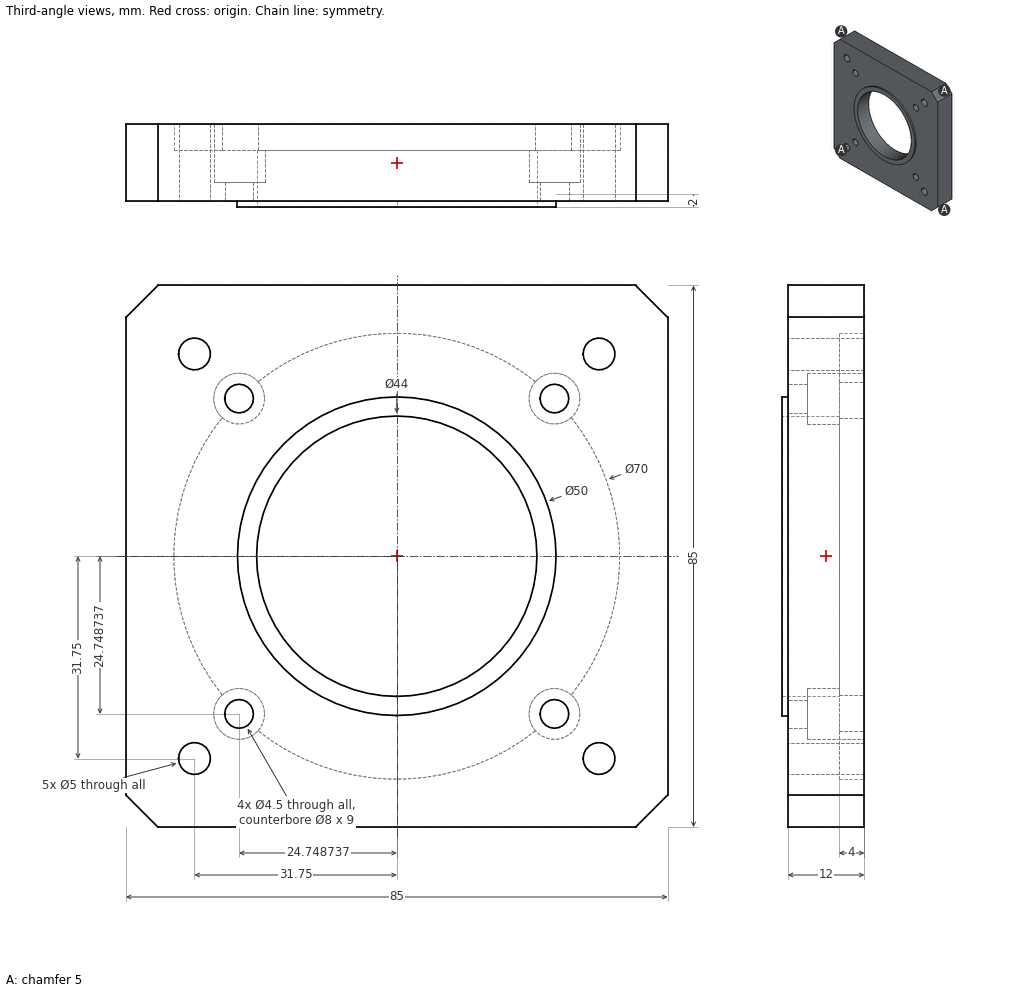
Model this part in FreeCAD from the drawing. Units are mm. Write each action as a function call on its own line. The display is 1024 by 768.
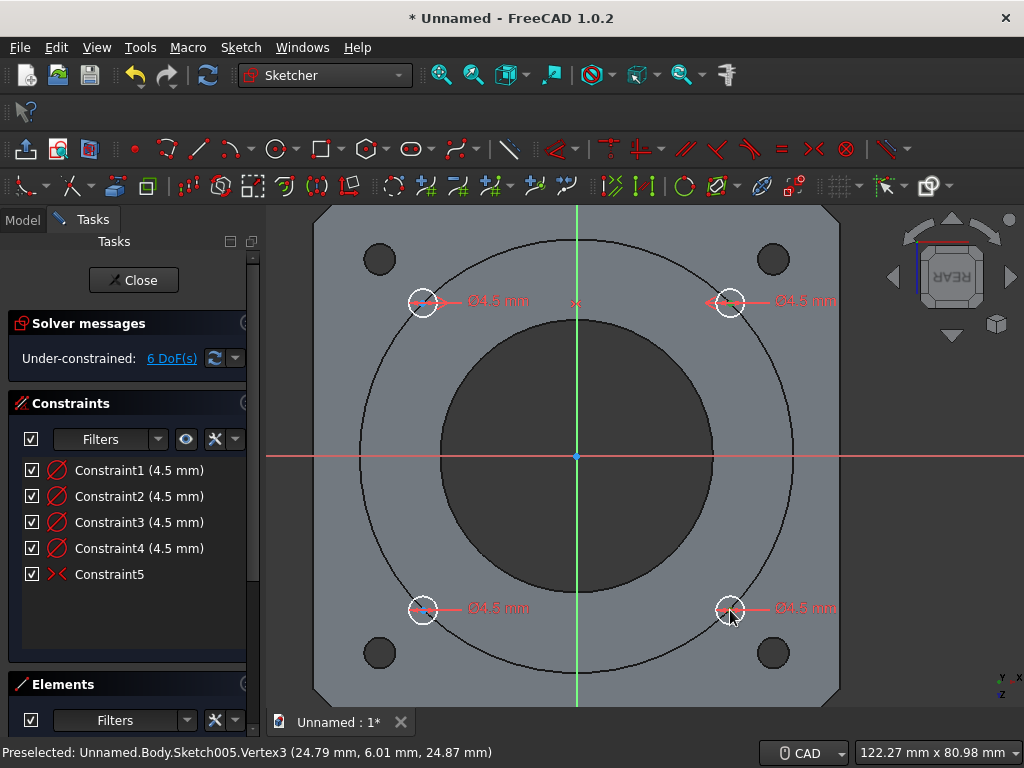
click(334, 456)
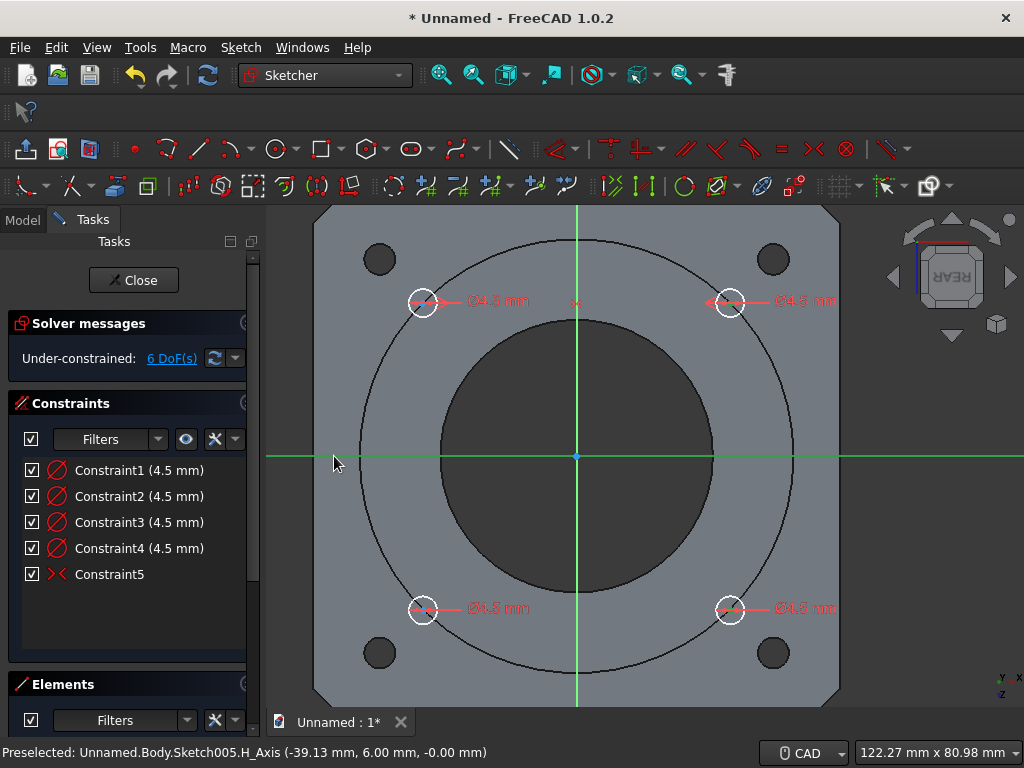
key(s)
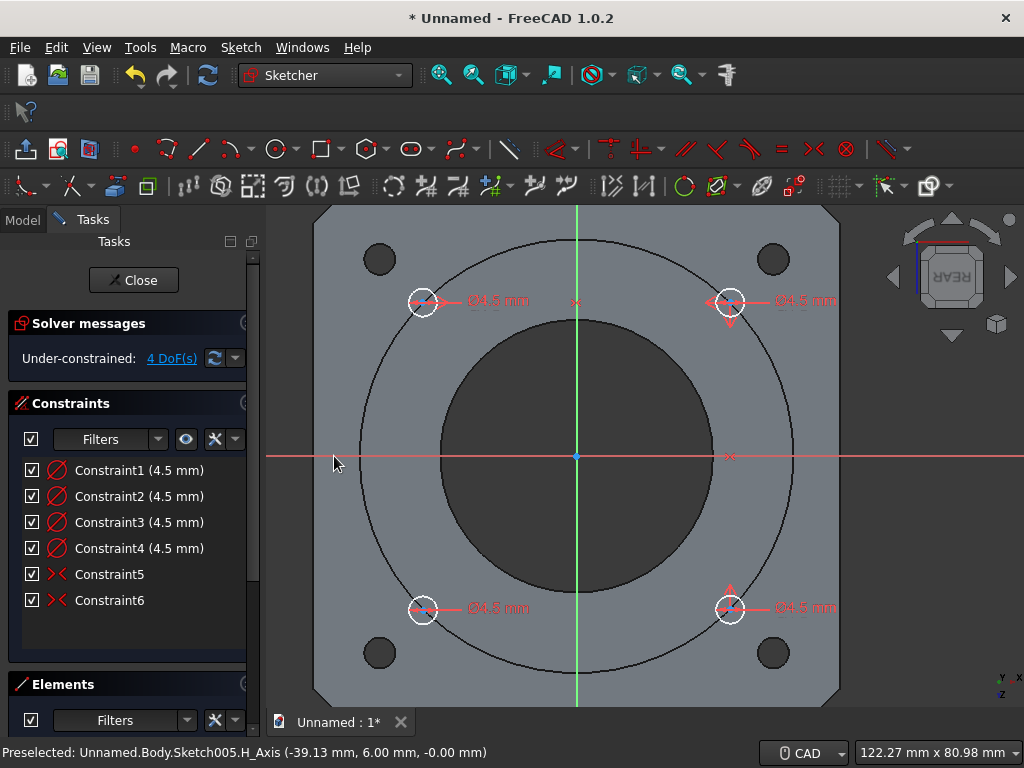
click(423, 303)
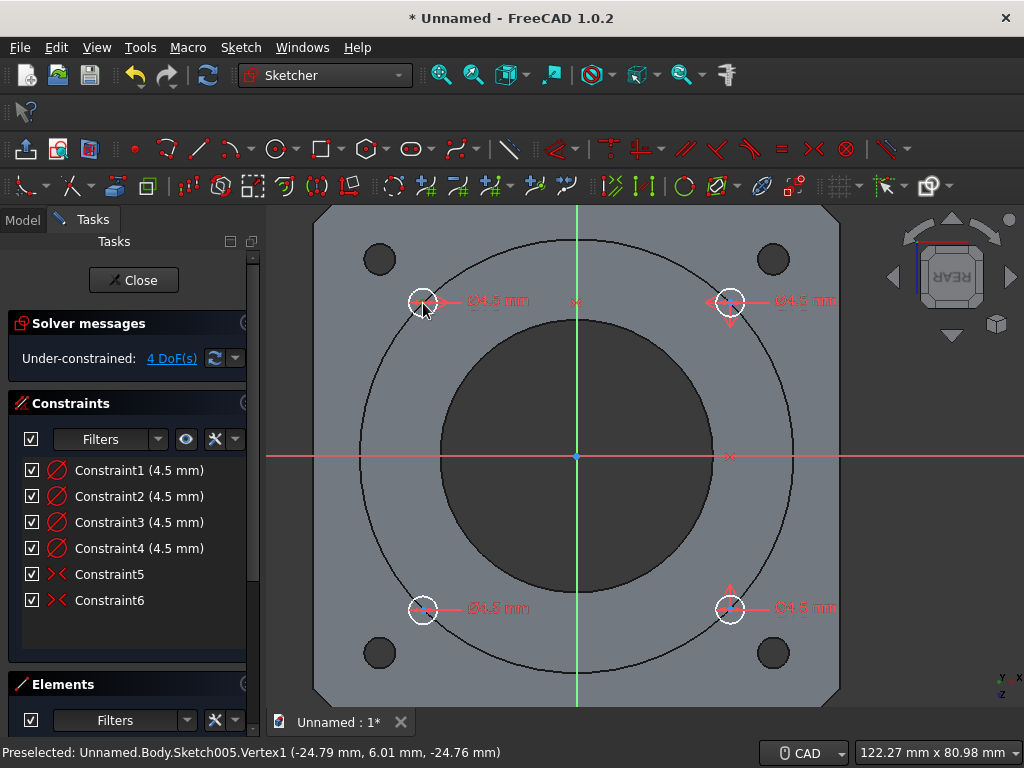
click(423, 610)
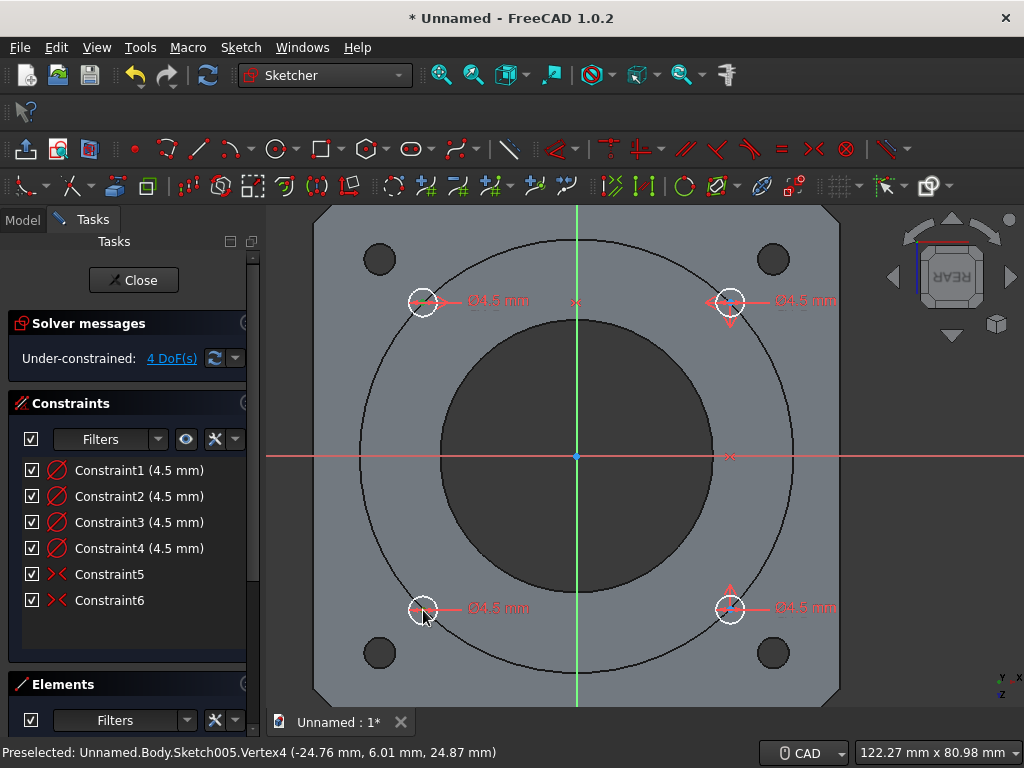
click(334, 456)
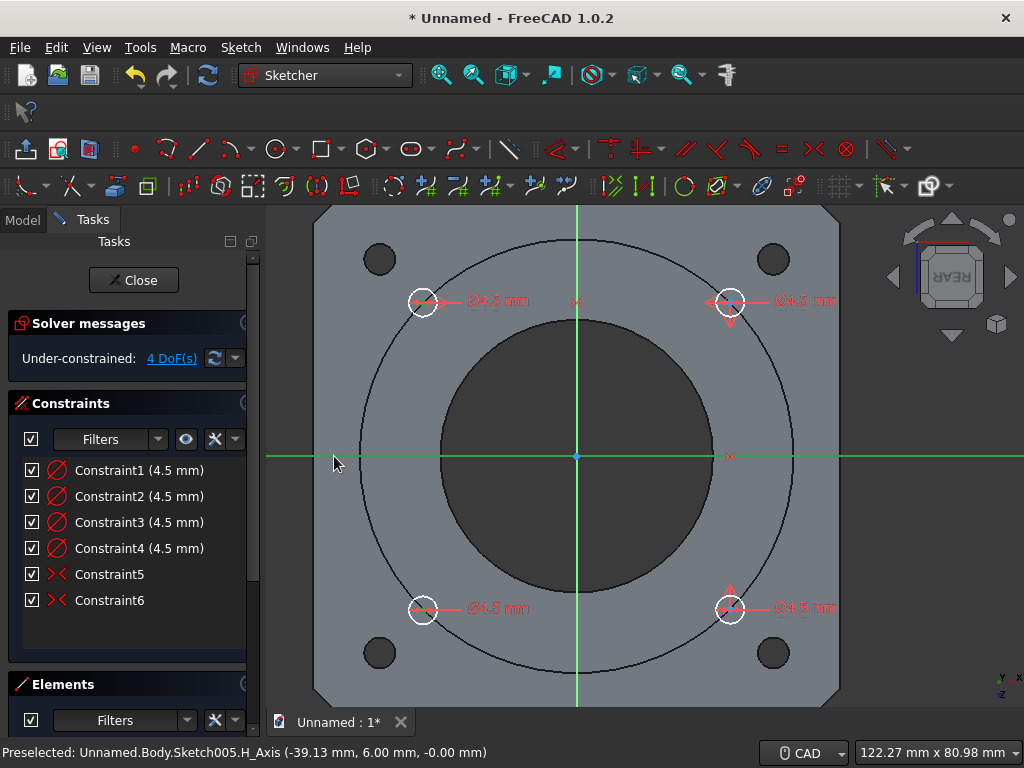
key(s)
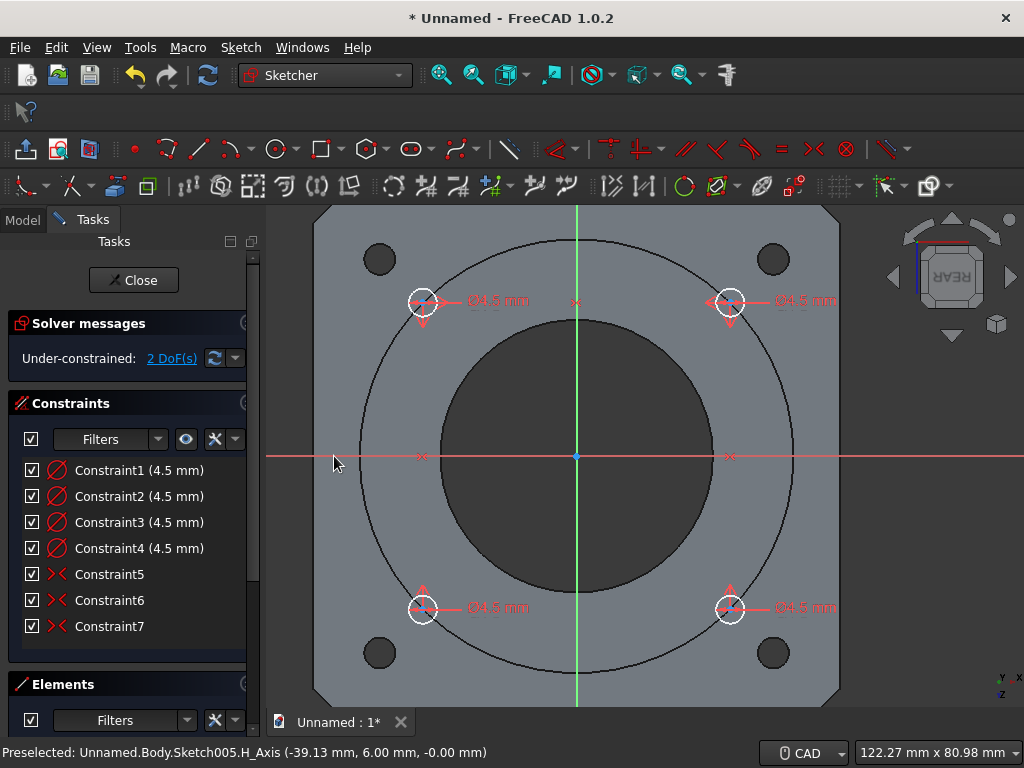
click(556, 150)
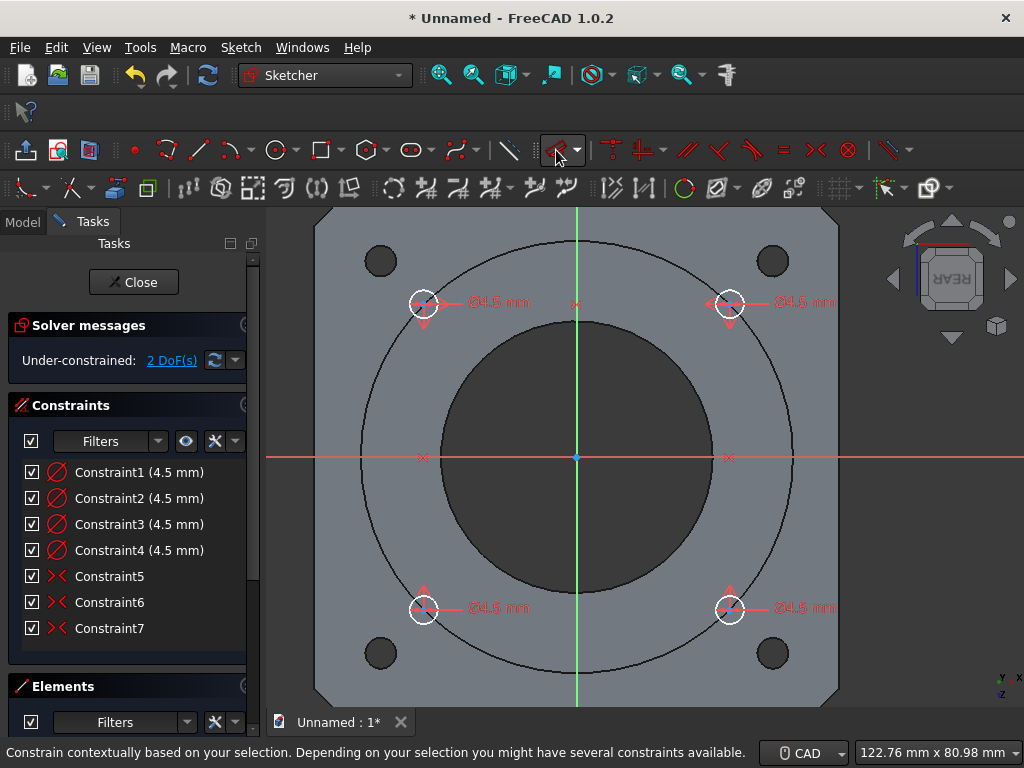
click(424, 304)
click(500, 270)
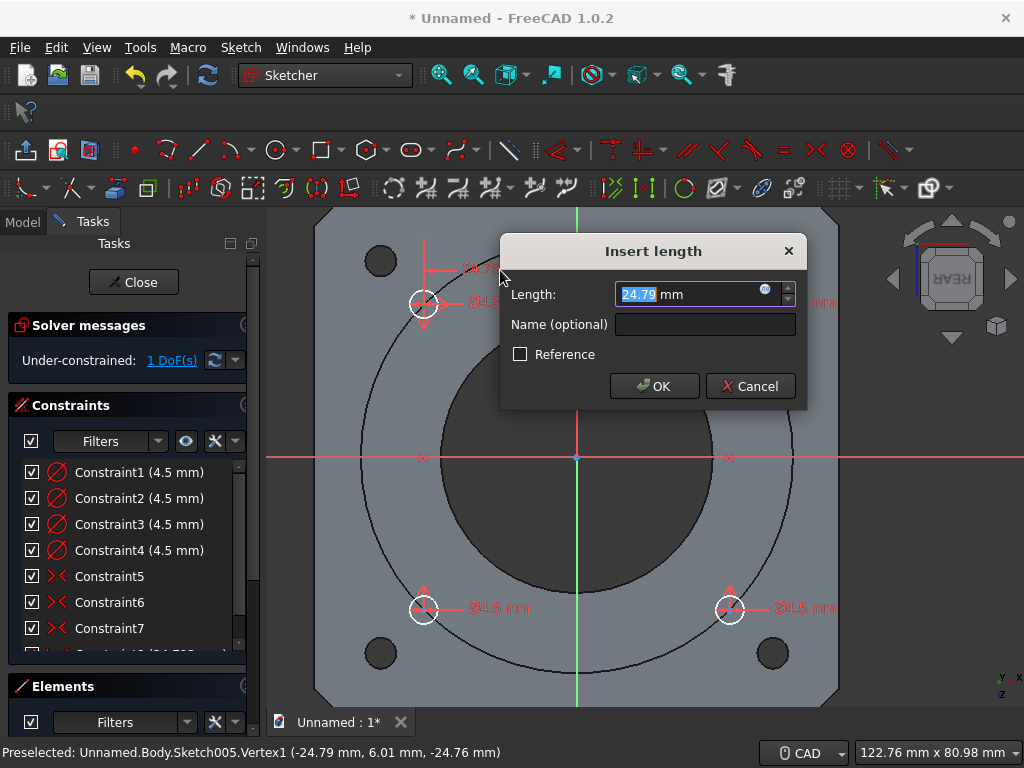
text(24.748737)
key(Return)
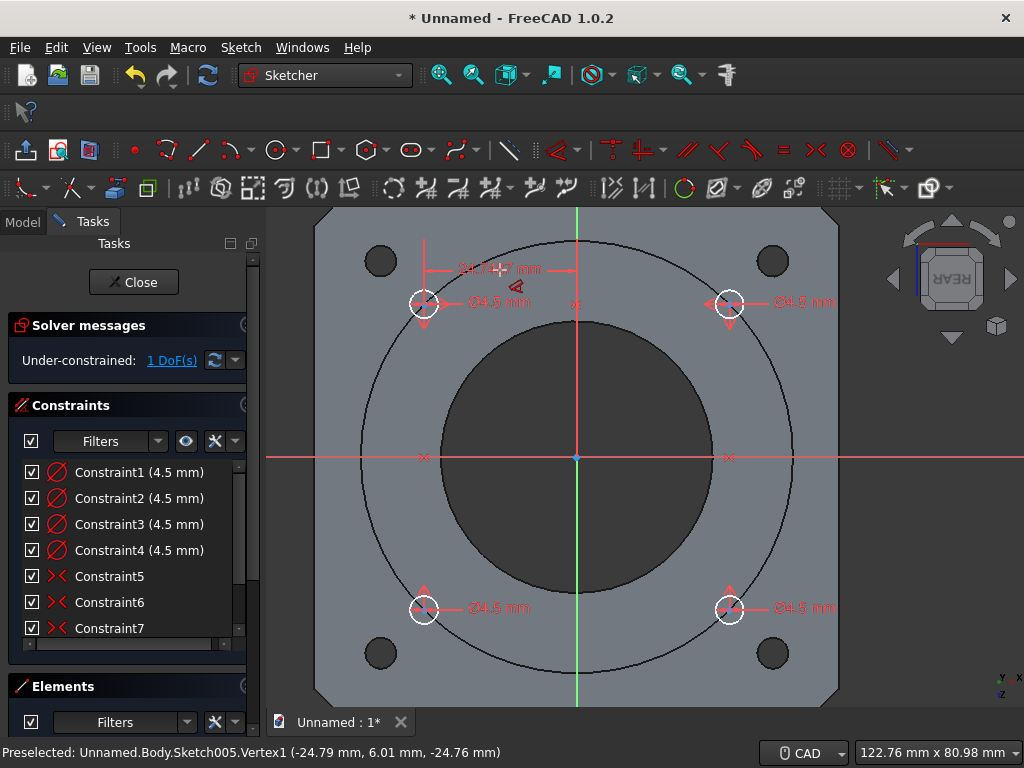
click(424, 304)
click(390, 381)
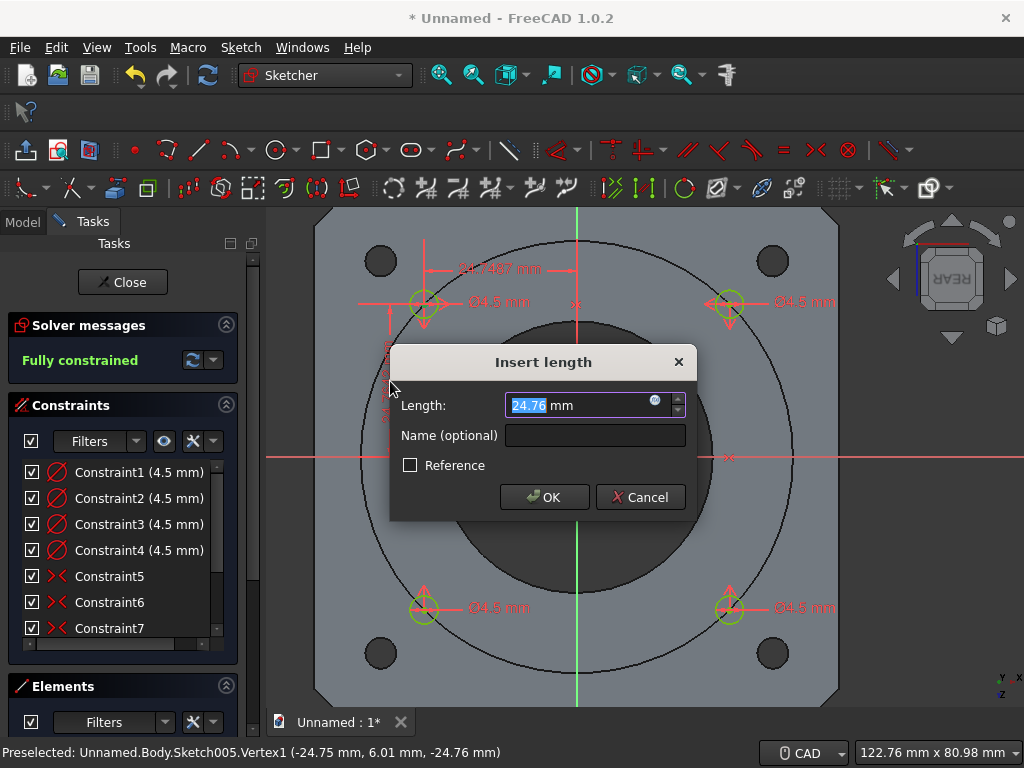
text(24.748737)
key(Return)
key(Escape)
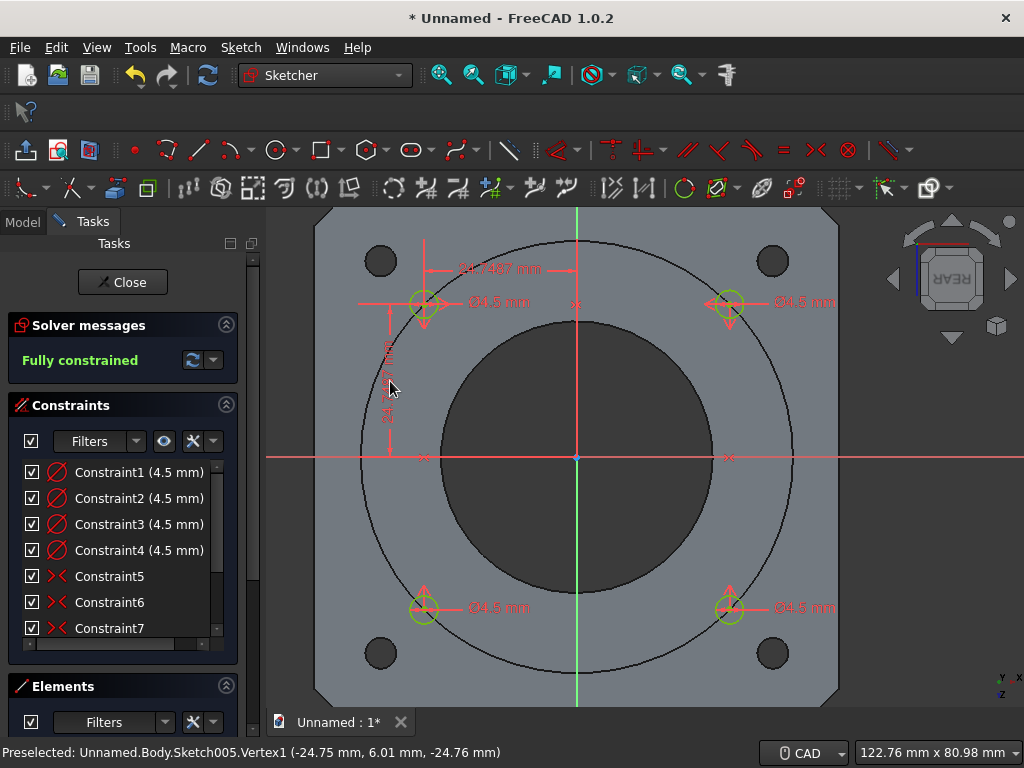
click(123, 282)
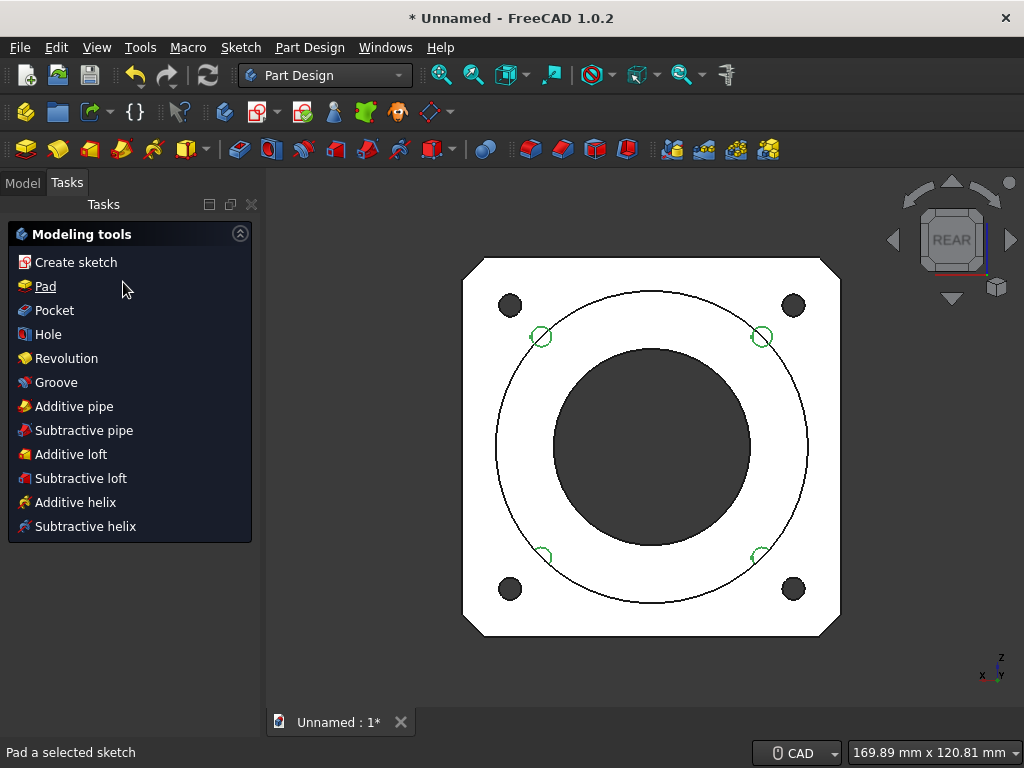
click(272, 150)